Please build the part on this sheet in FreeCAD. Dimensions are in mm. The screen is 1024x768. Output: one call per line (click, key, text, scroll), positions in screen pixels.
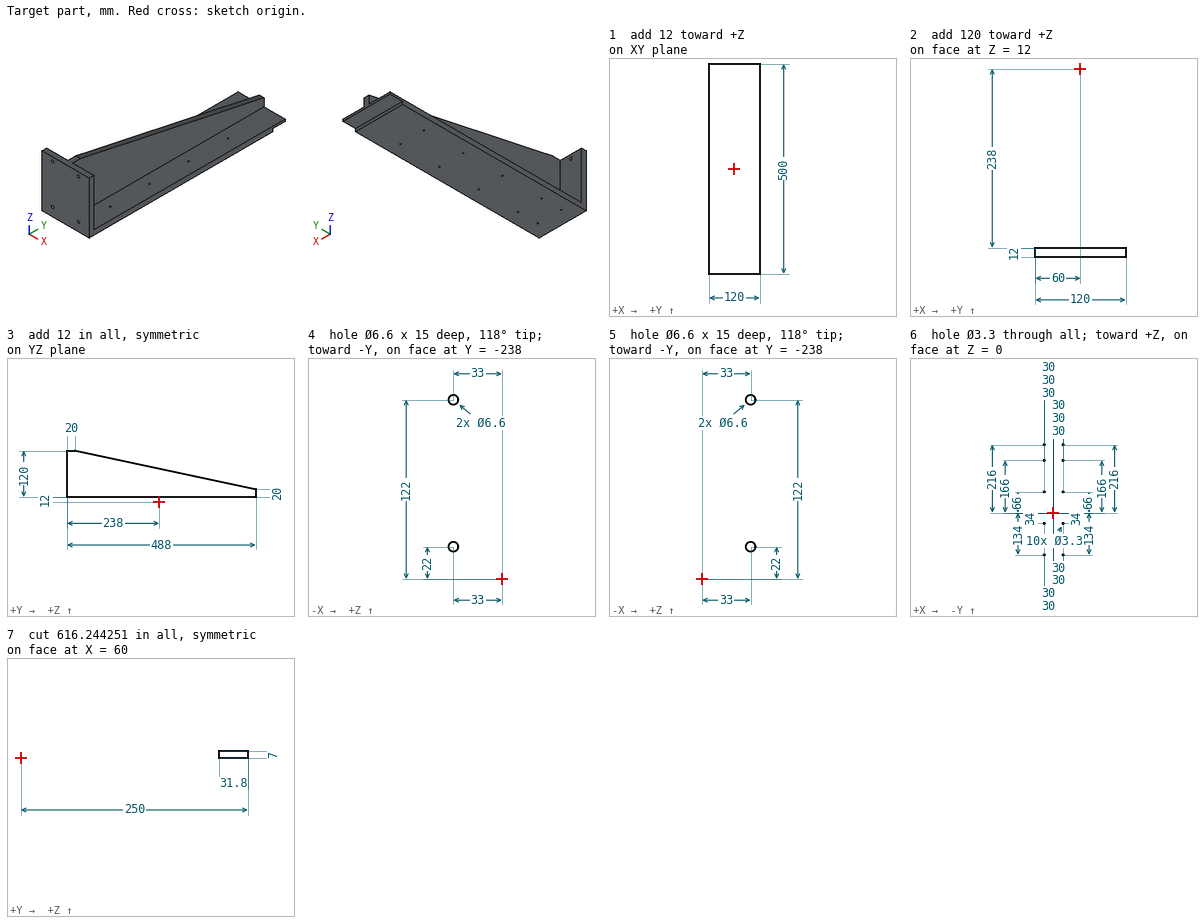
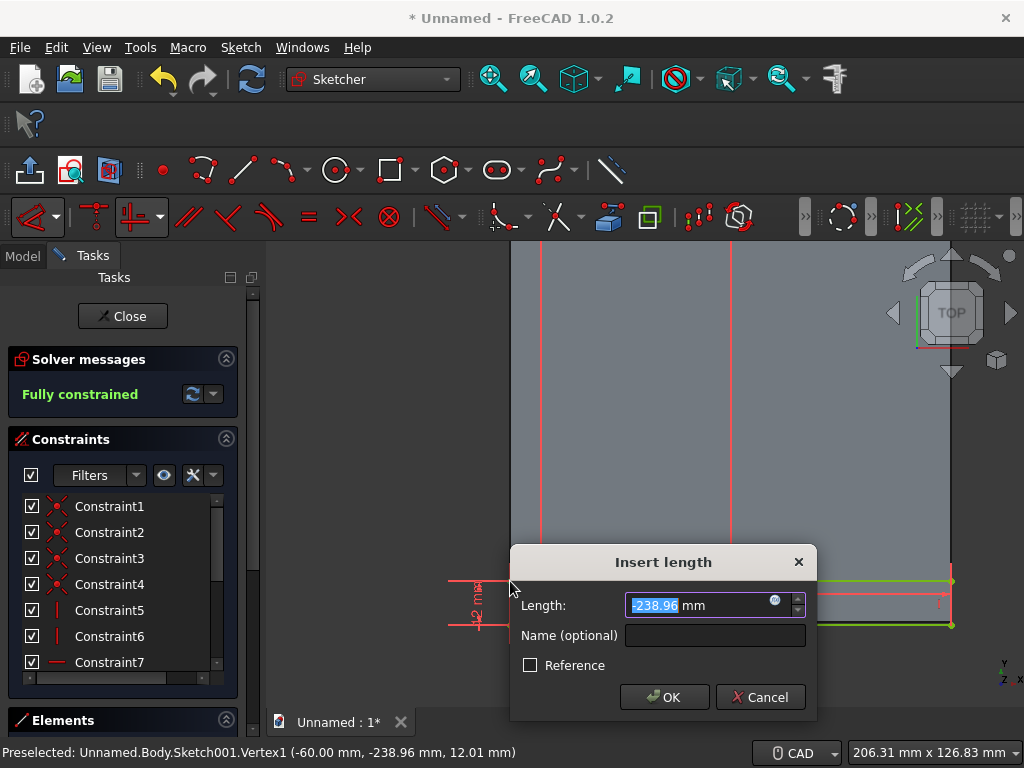
text(-238)
key(Return)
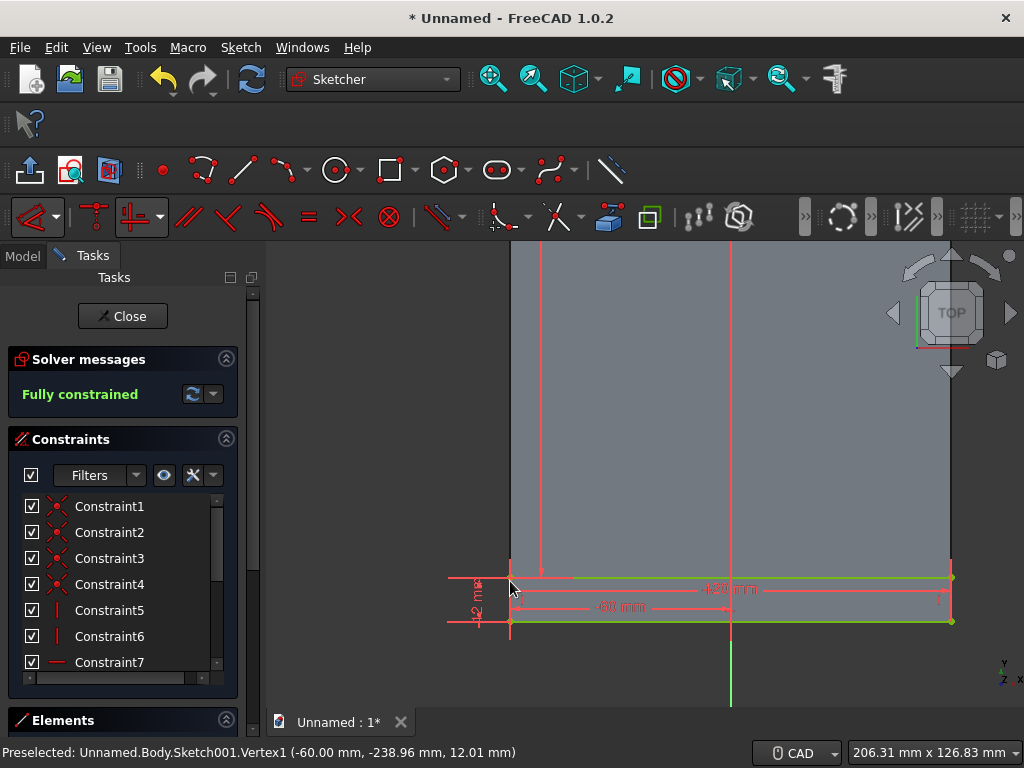
click(123, 316)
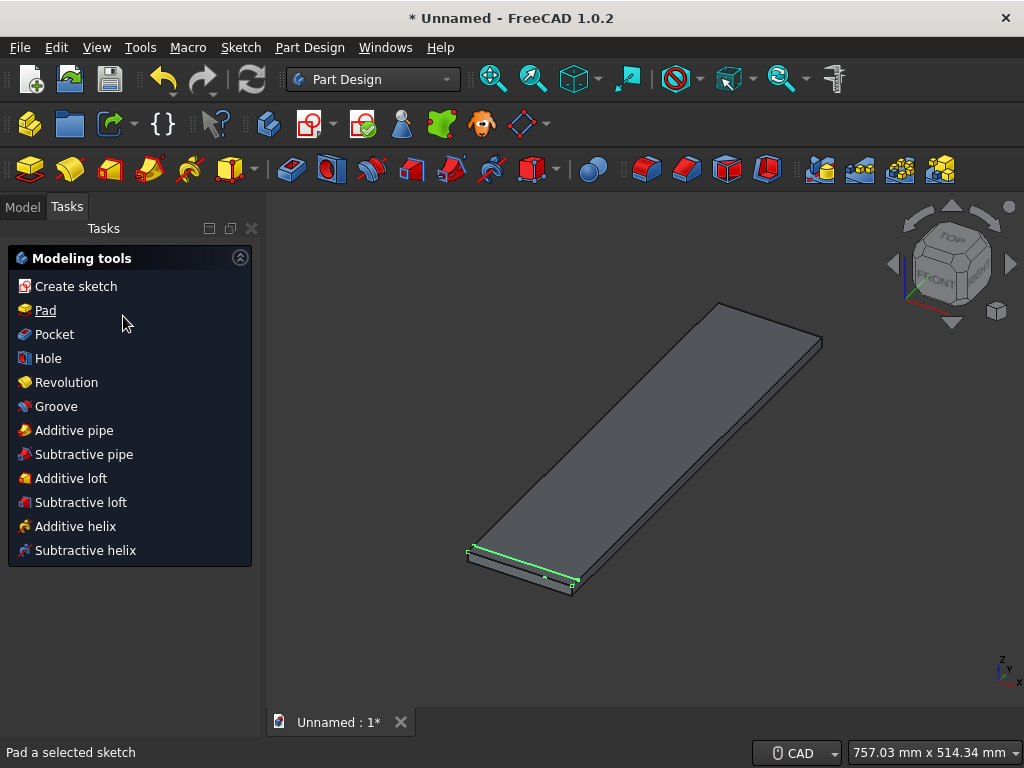
click(30, 170)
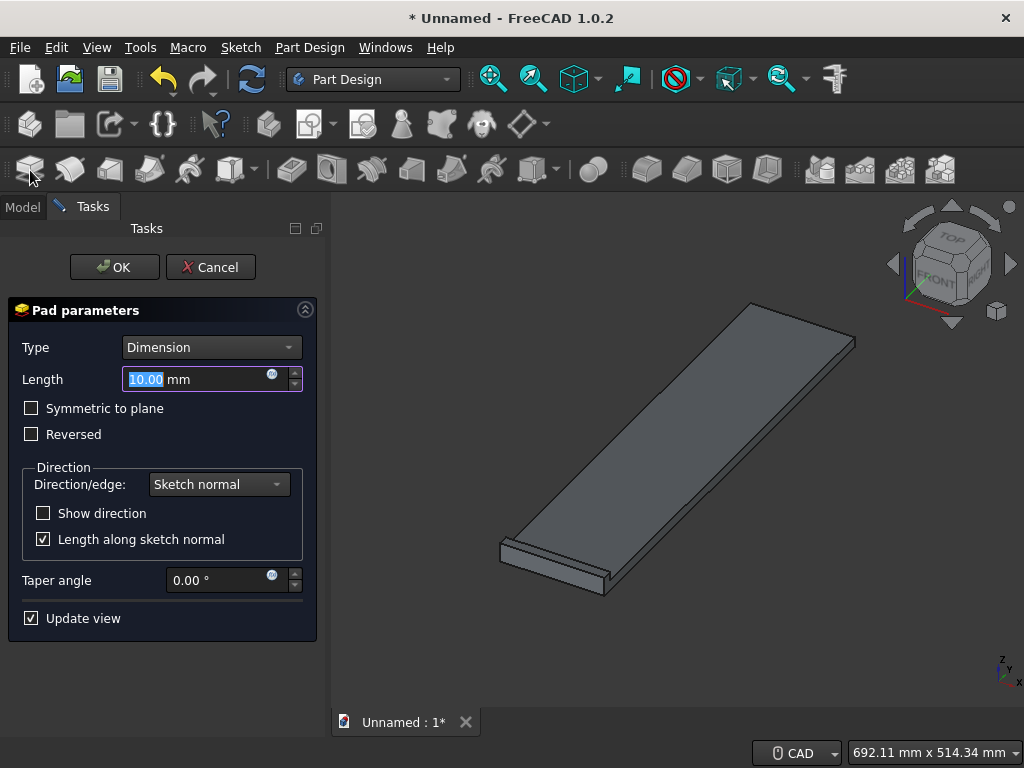
text(120)
key(Tab)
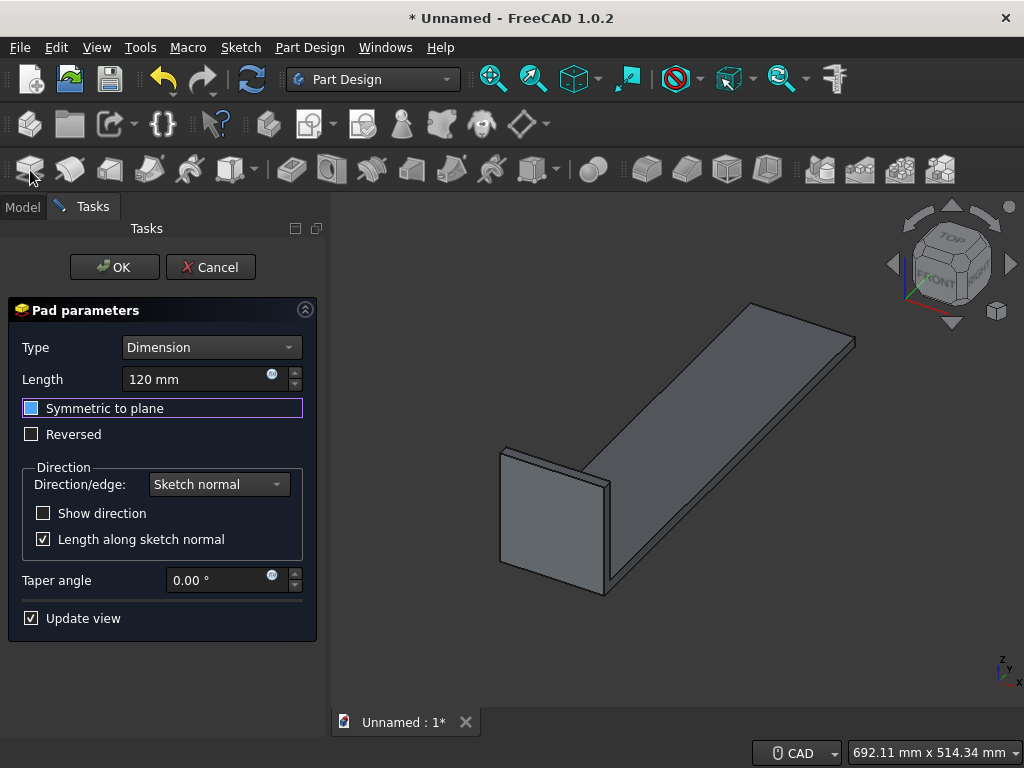
click(115, 267)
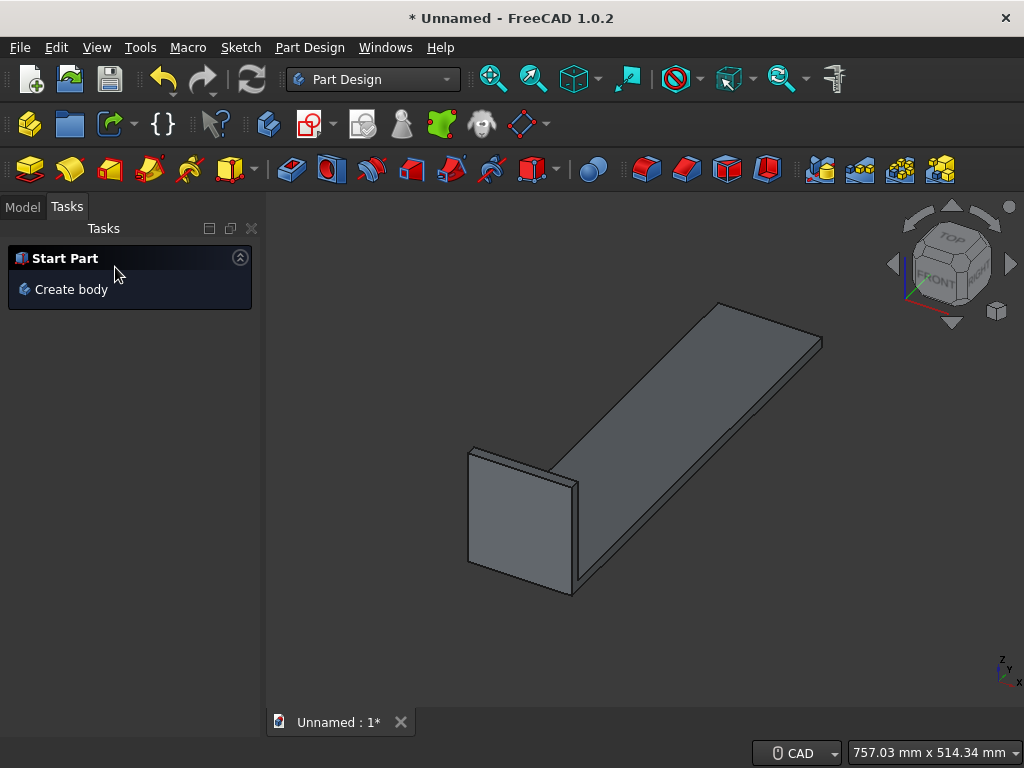
click(310, 124)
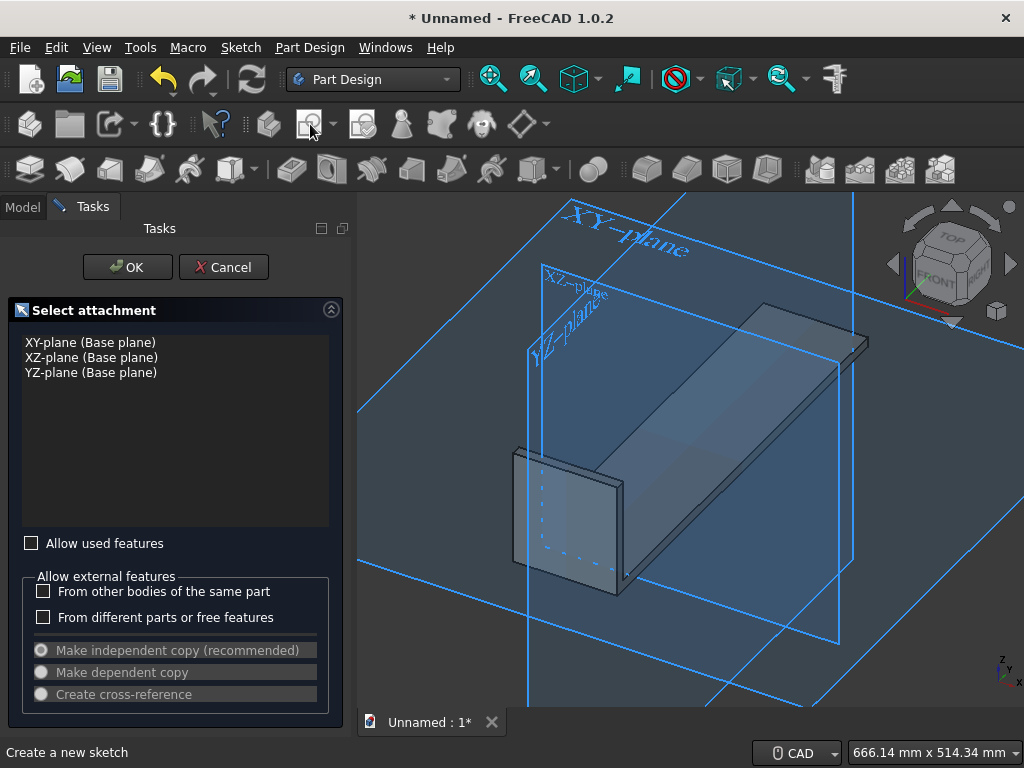
click(82, 372)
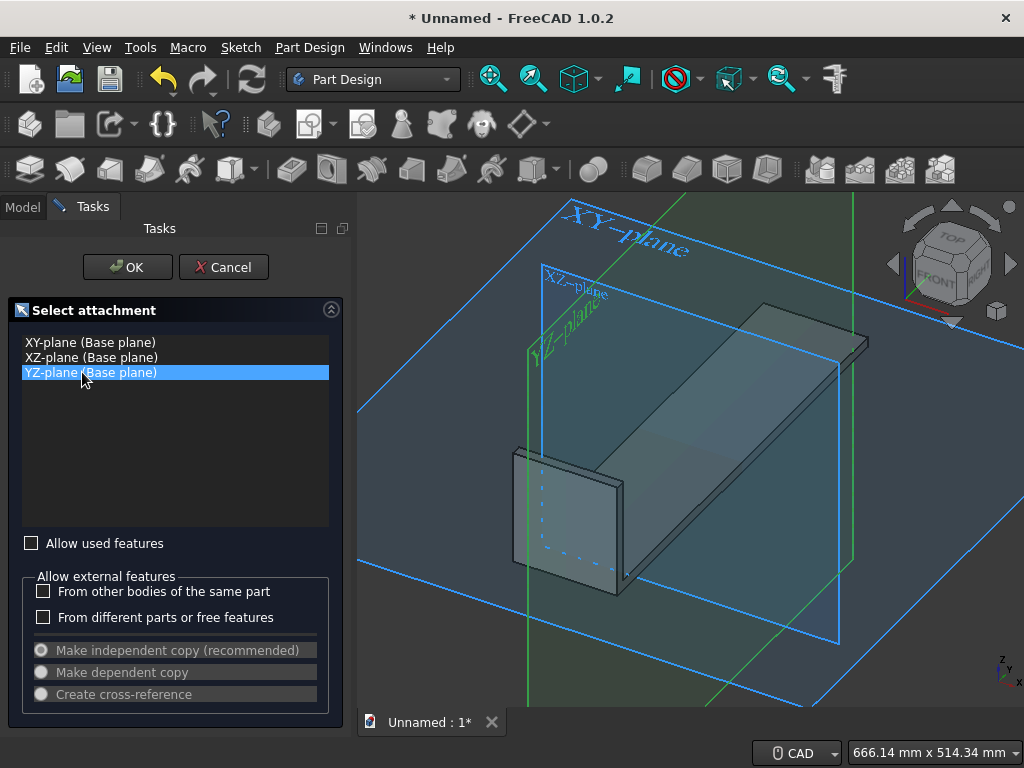
click(128, 267)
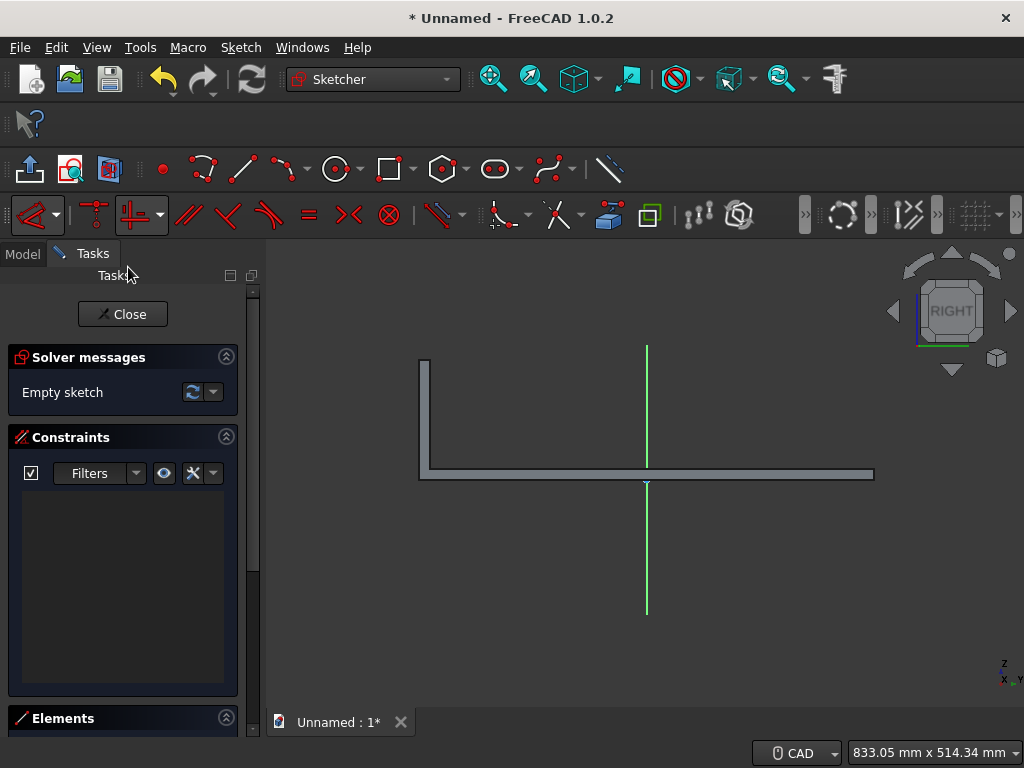
click(110, 170)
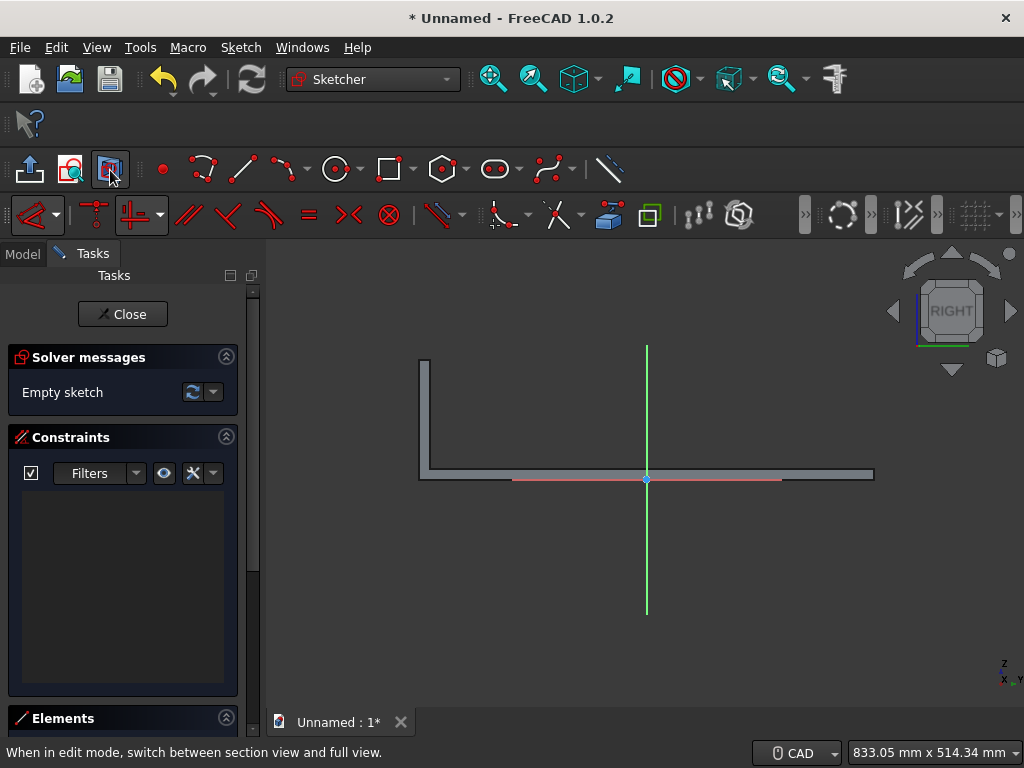
scroll(294, 679, down, 1)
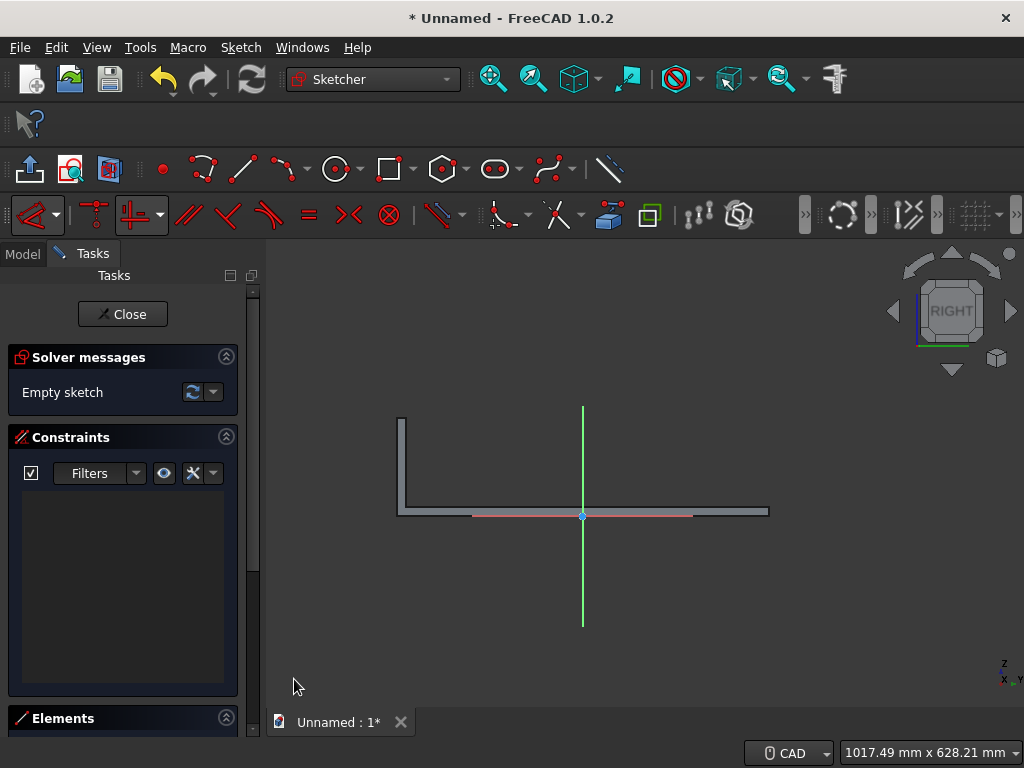
click(204, 170)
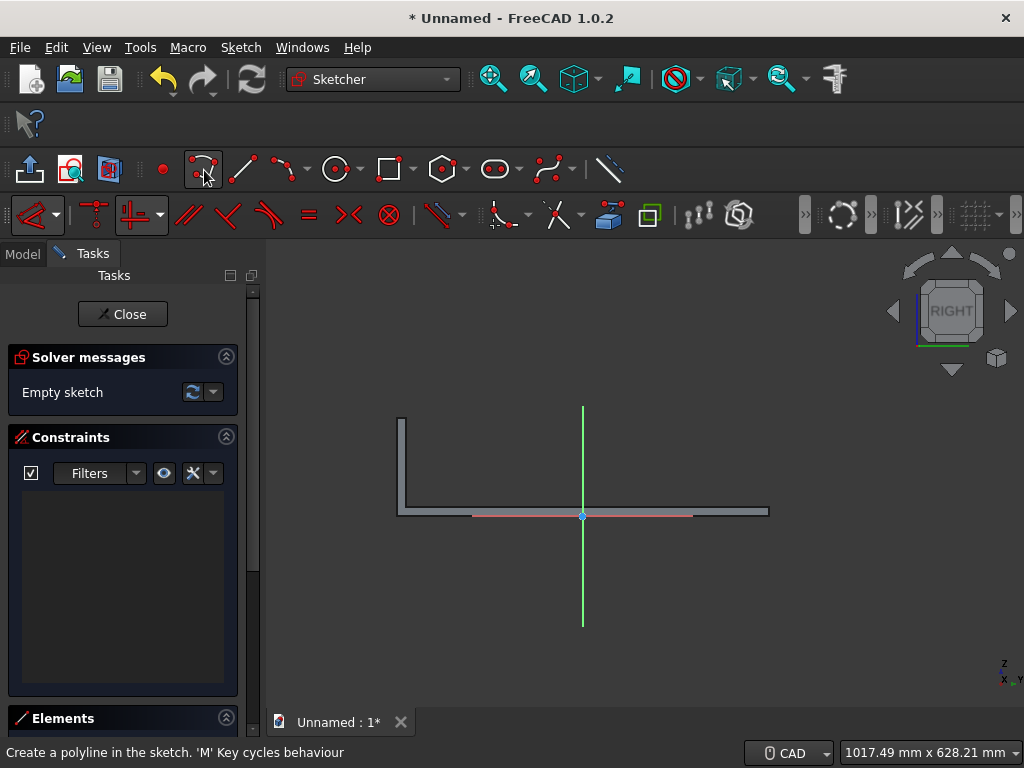
scroll(406, 507, up, 3)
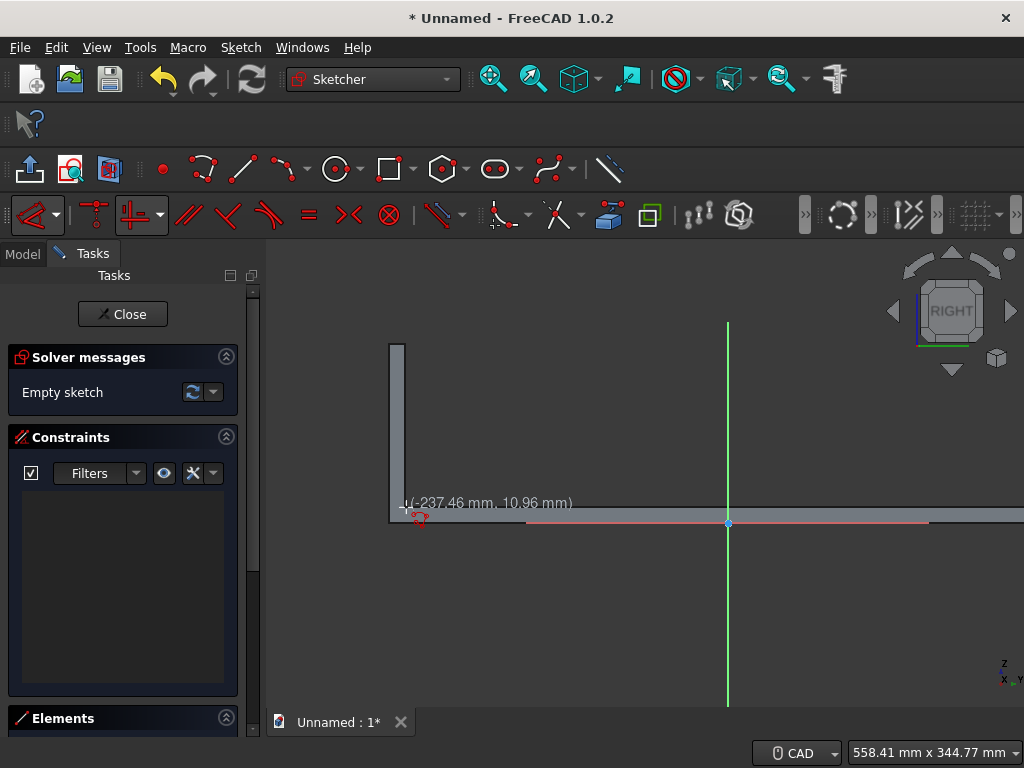
click(405, 507)